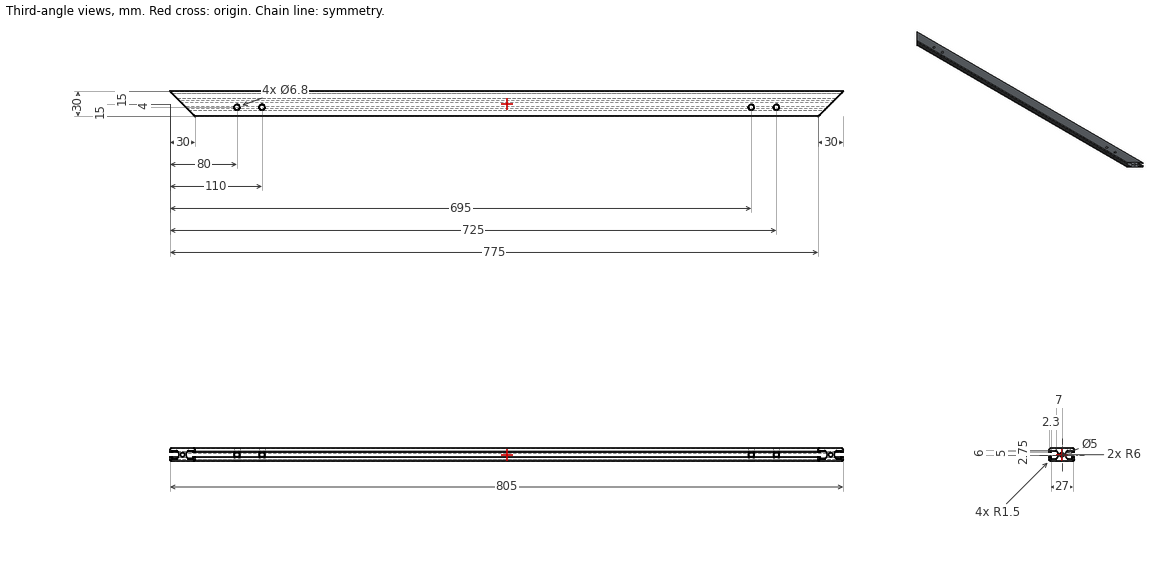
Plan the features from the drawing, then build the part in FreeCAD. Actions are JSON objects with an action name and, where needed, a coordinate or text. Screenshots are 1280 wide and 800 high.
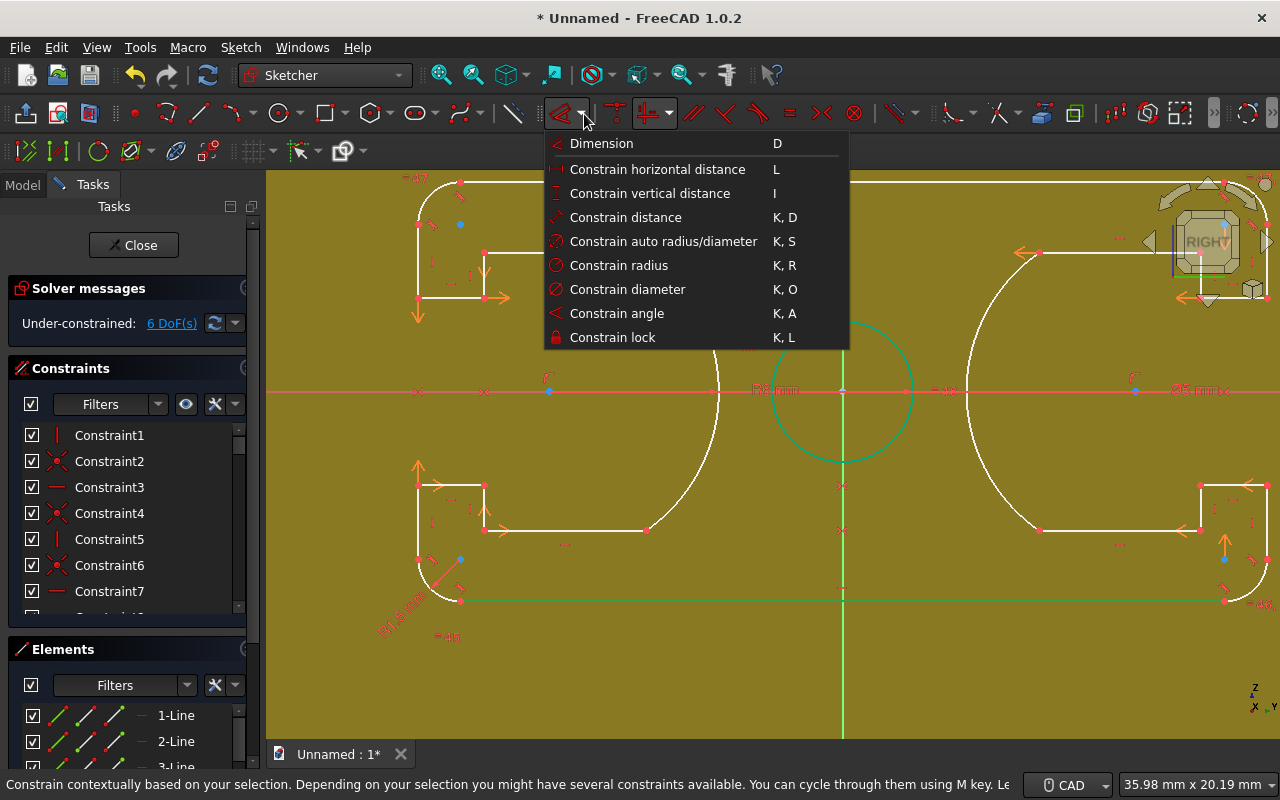
{"action": "left_click", "coordinate": [697, 169]}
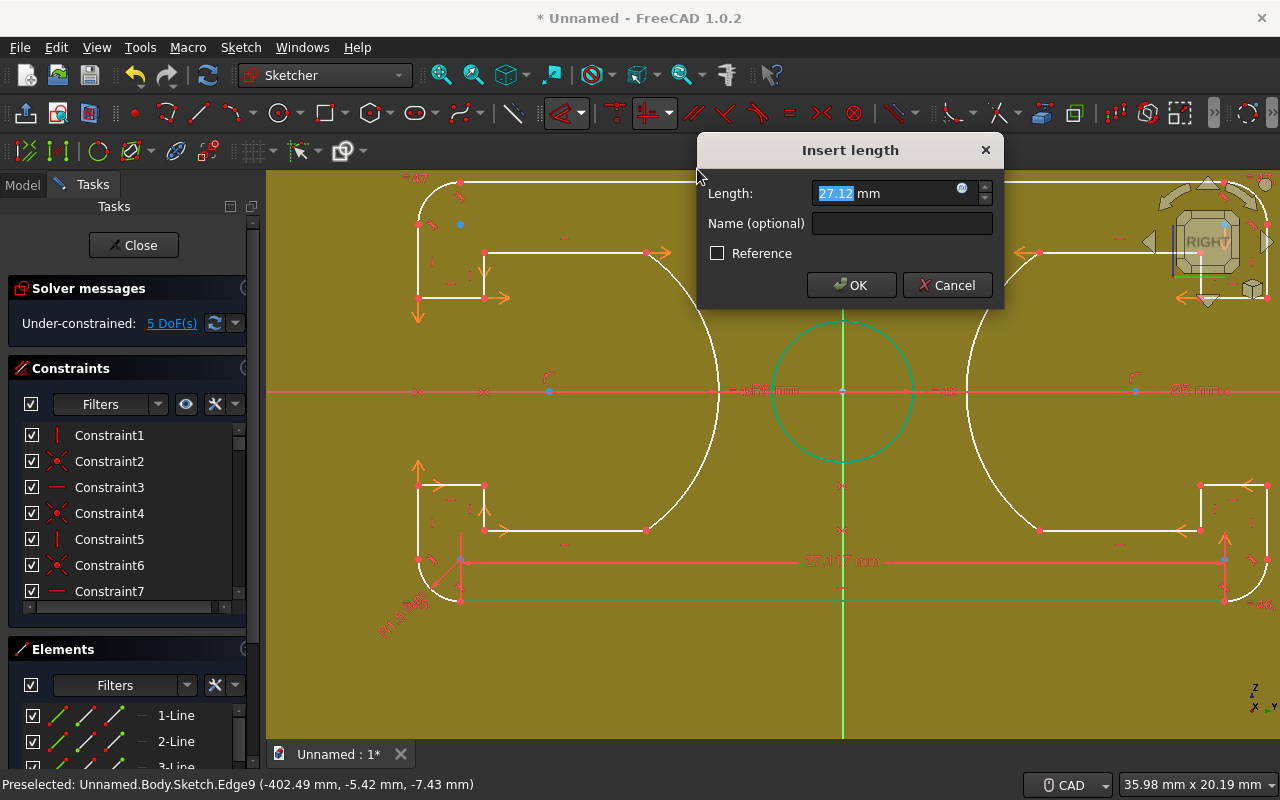
{"action": "type", "text": "27"}
{"action": "key", "text": "Return"}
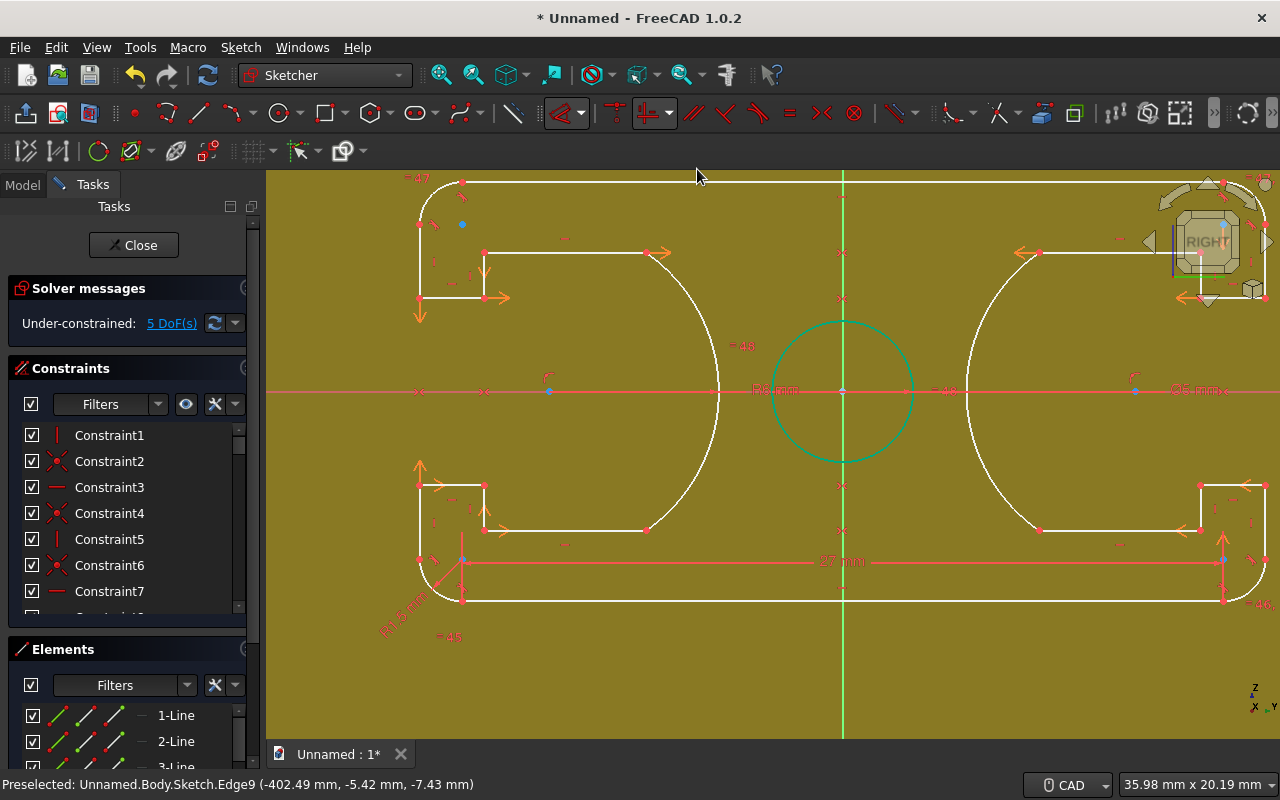
{"action": "left_click", "coordinate": [420, 224]}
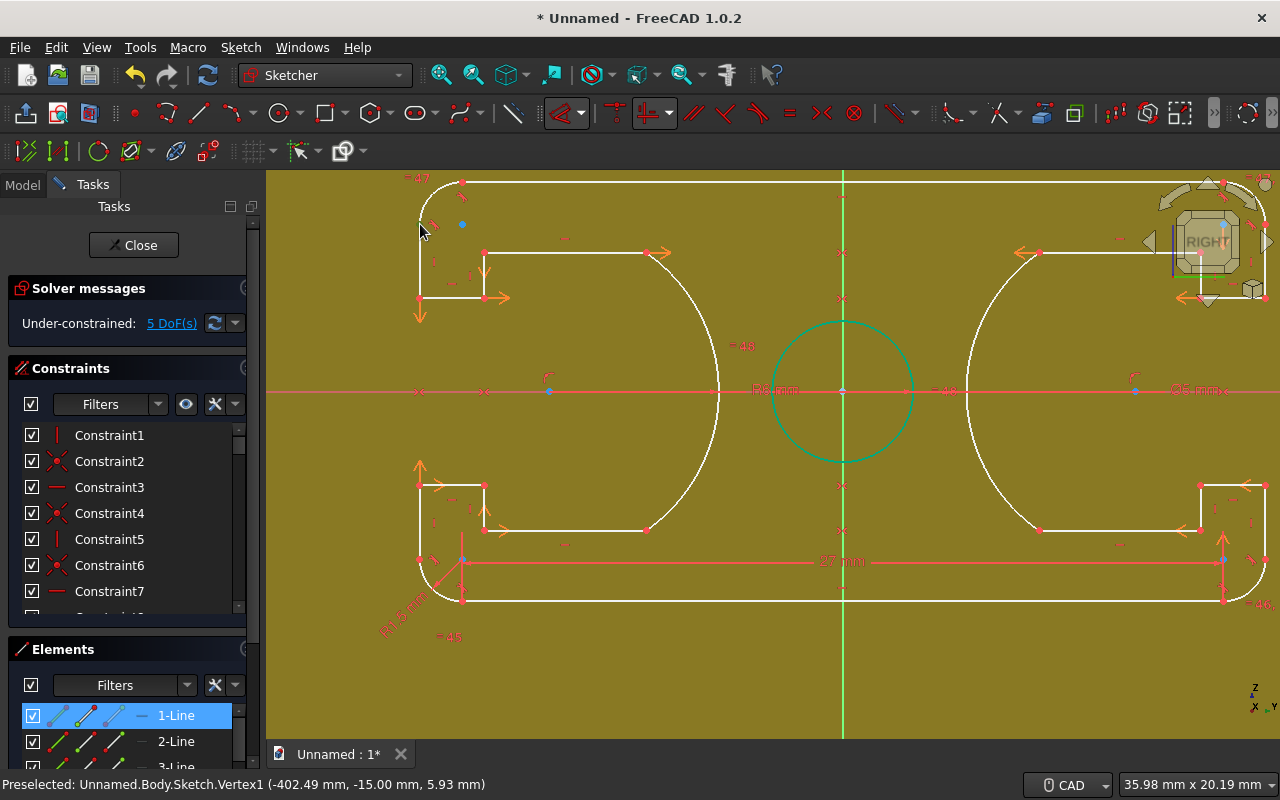
{"action": "left_click", "coordinate": [584, 114]}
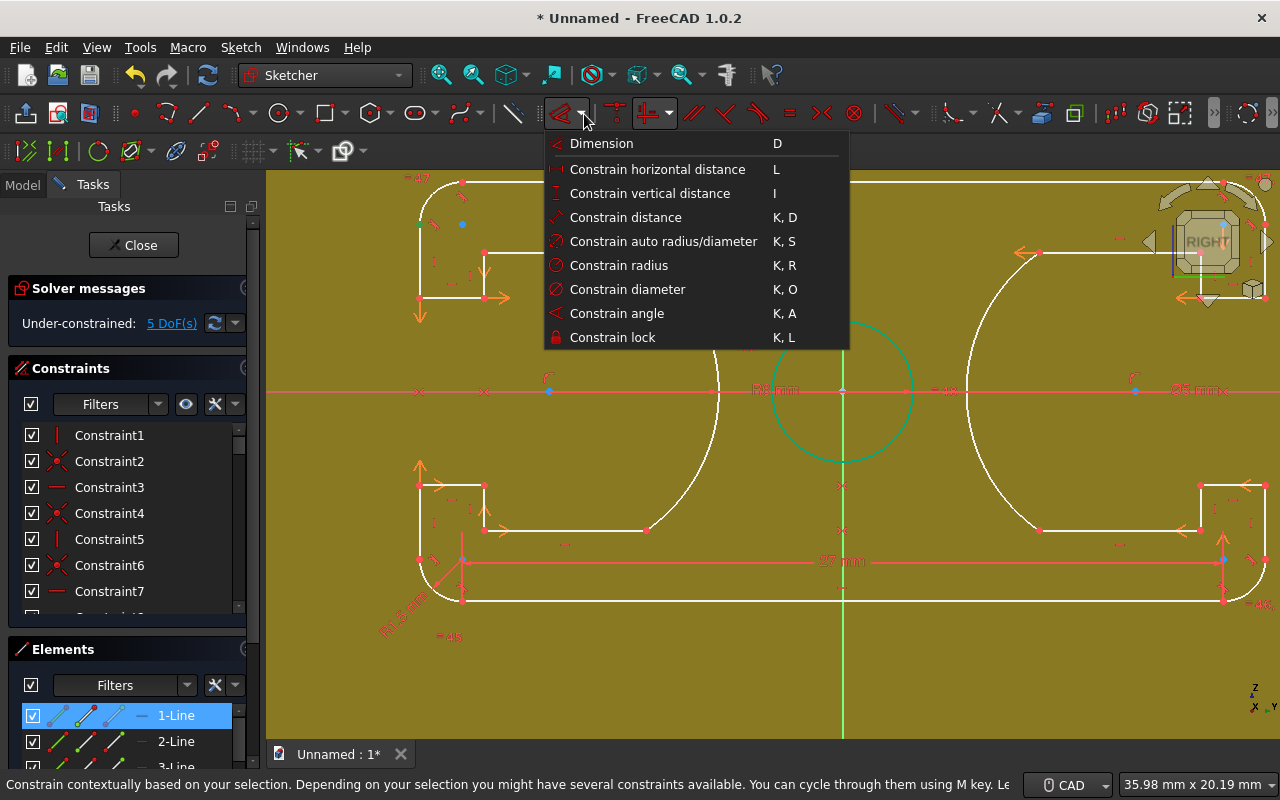
{"action": "left_click", "coordinate": [697, 193]}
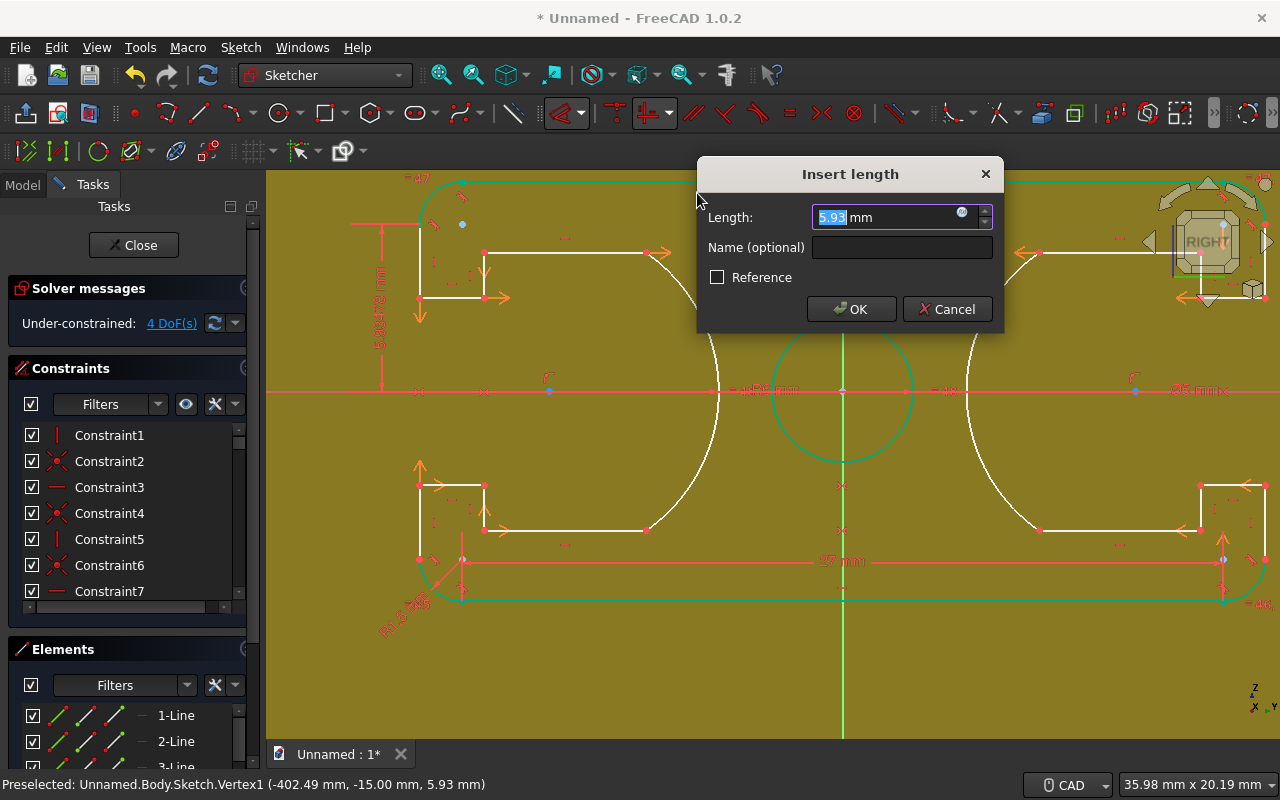
{"action": "type", "text": "6"}
{"action": "key", "text": "Return"}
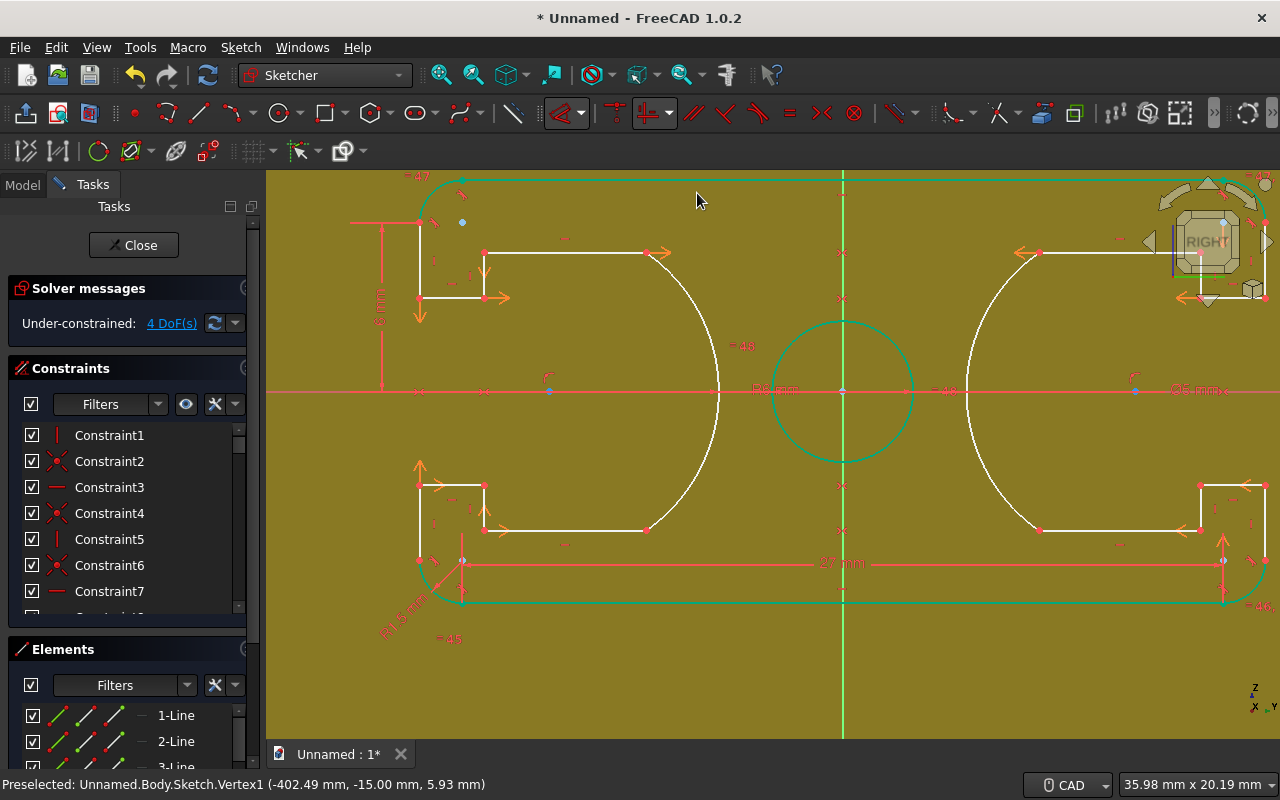
{"action": "left_click", "coordinate": [484, 253]}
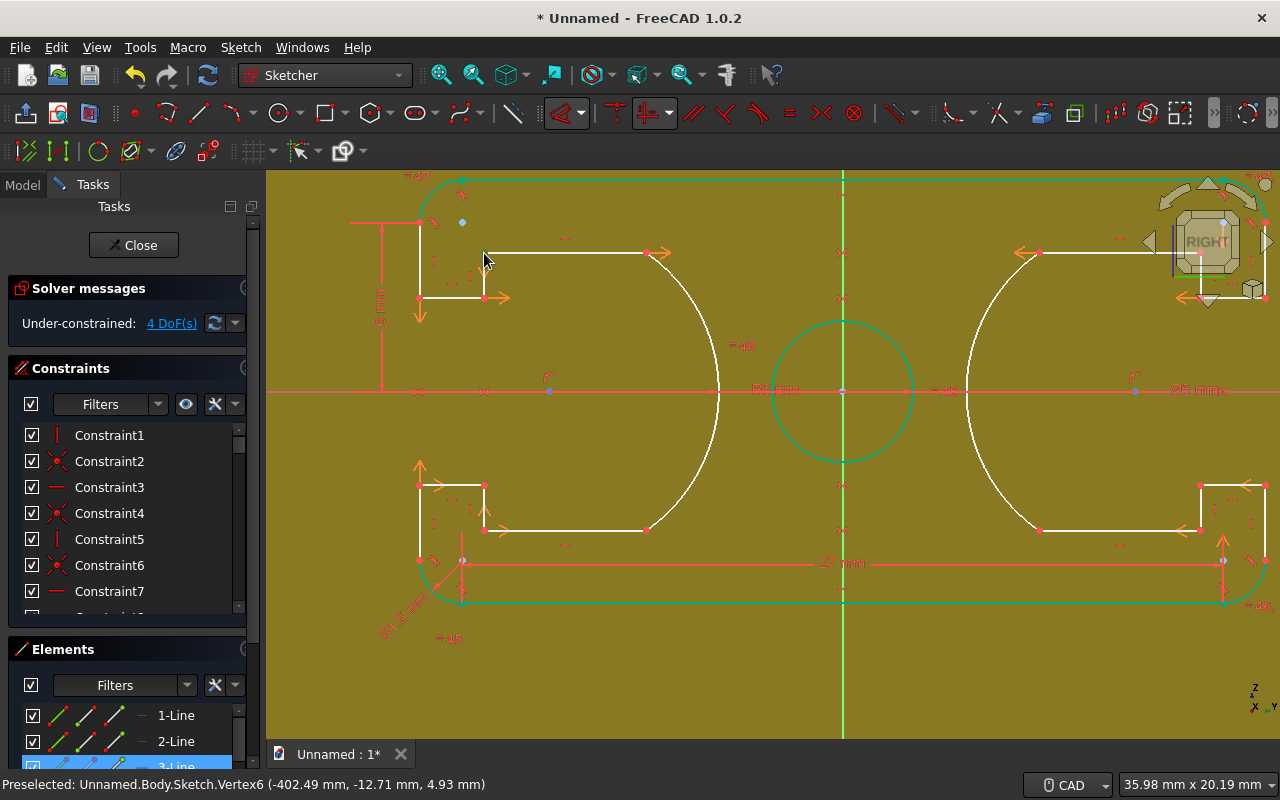
{"action": "left_click", "coordinate": [584, 114]}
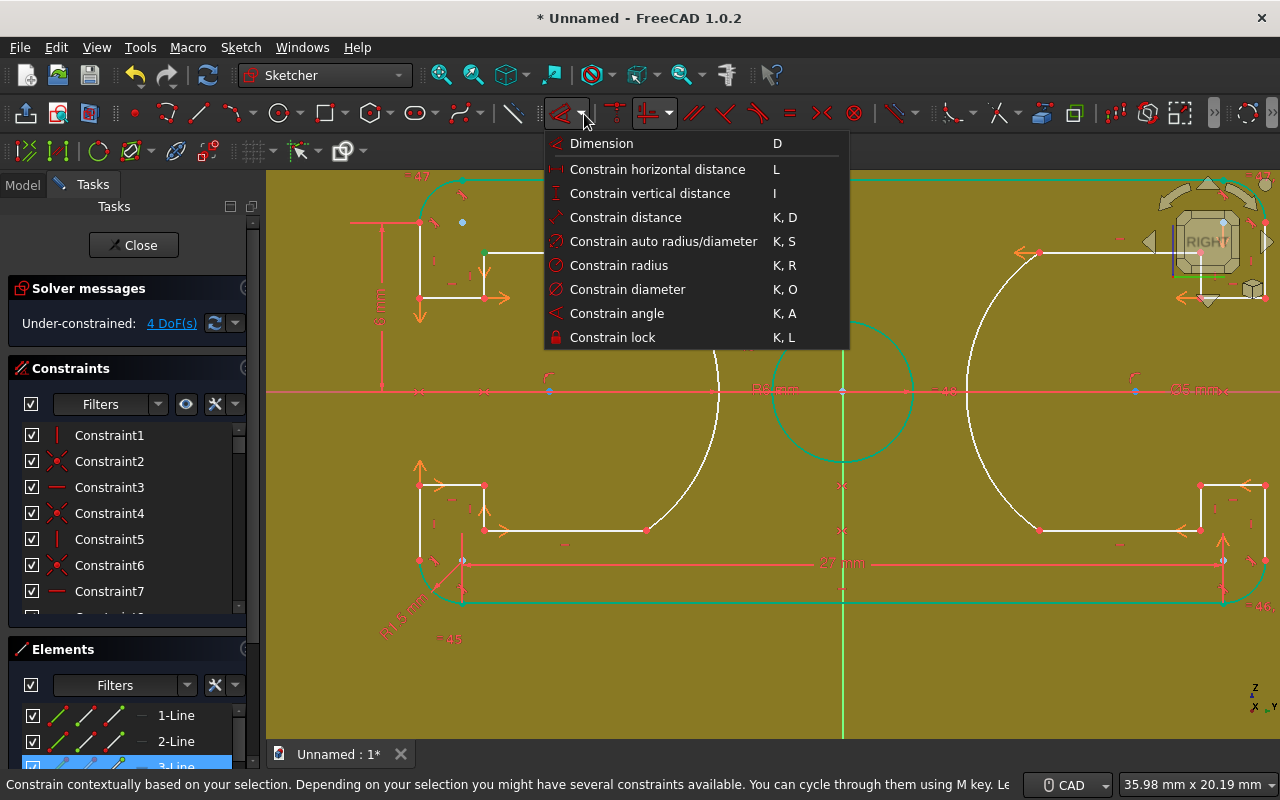
{"action": "left_click", "coordinate": [697, 193]}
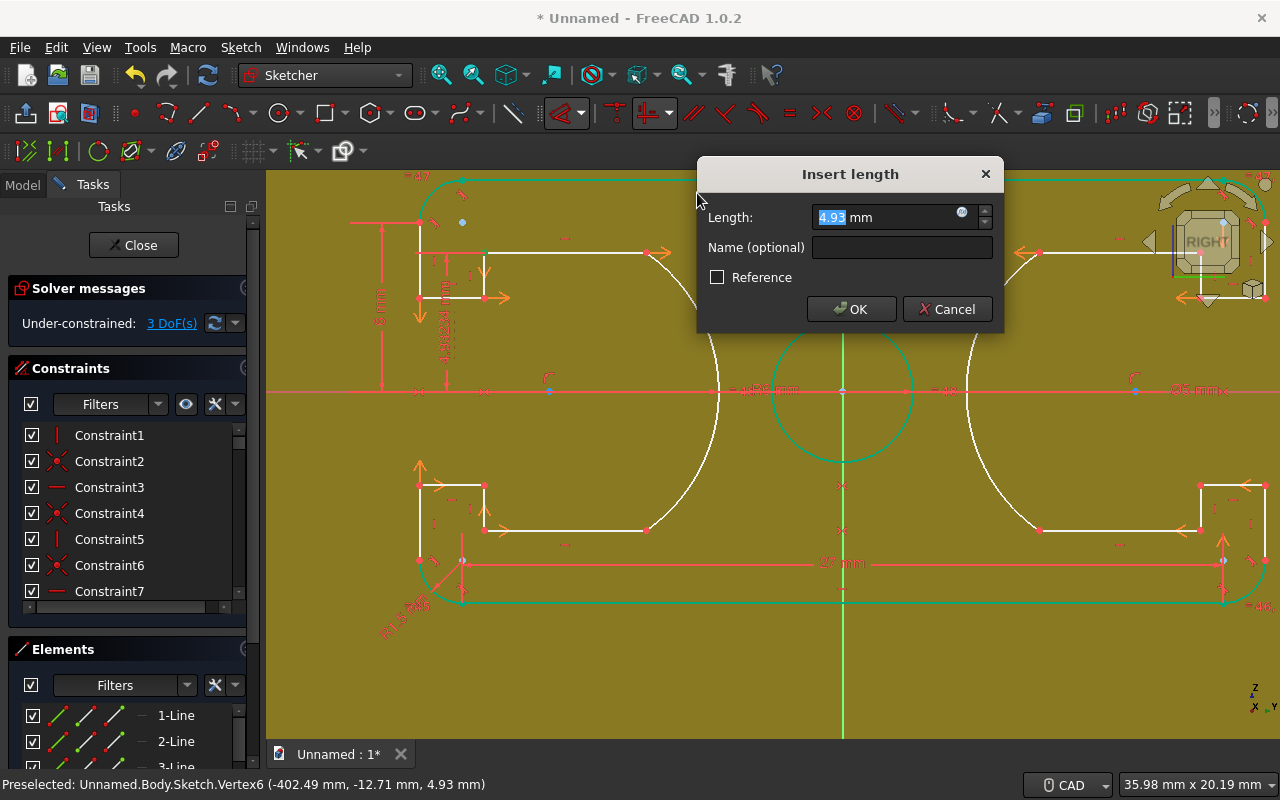
{"action": "type", "text": "5"}
{"action": "key", "text": "Return"}